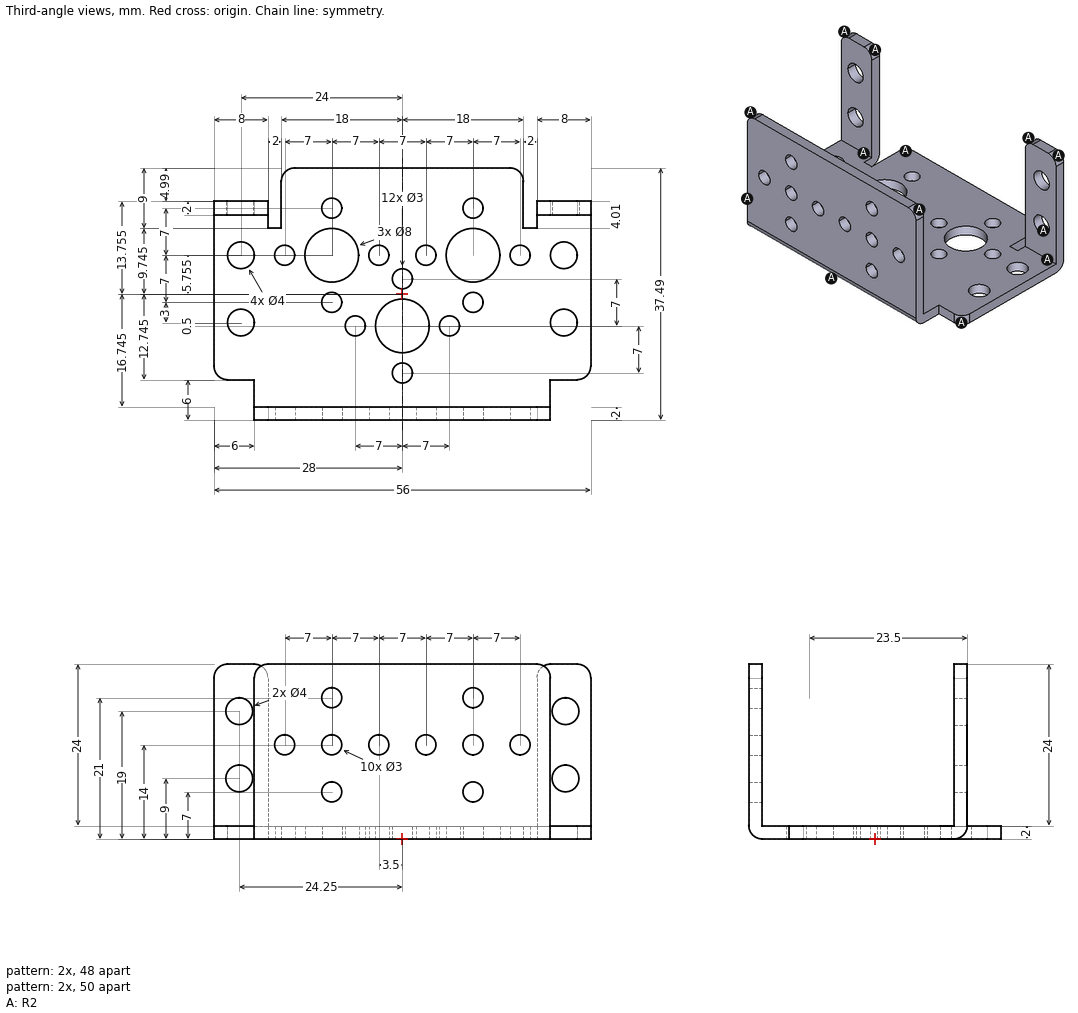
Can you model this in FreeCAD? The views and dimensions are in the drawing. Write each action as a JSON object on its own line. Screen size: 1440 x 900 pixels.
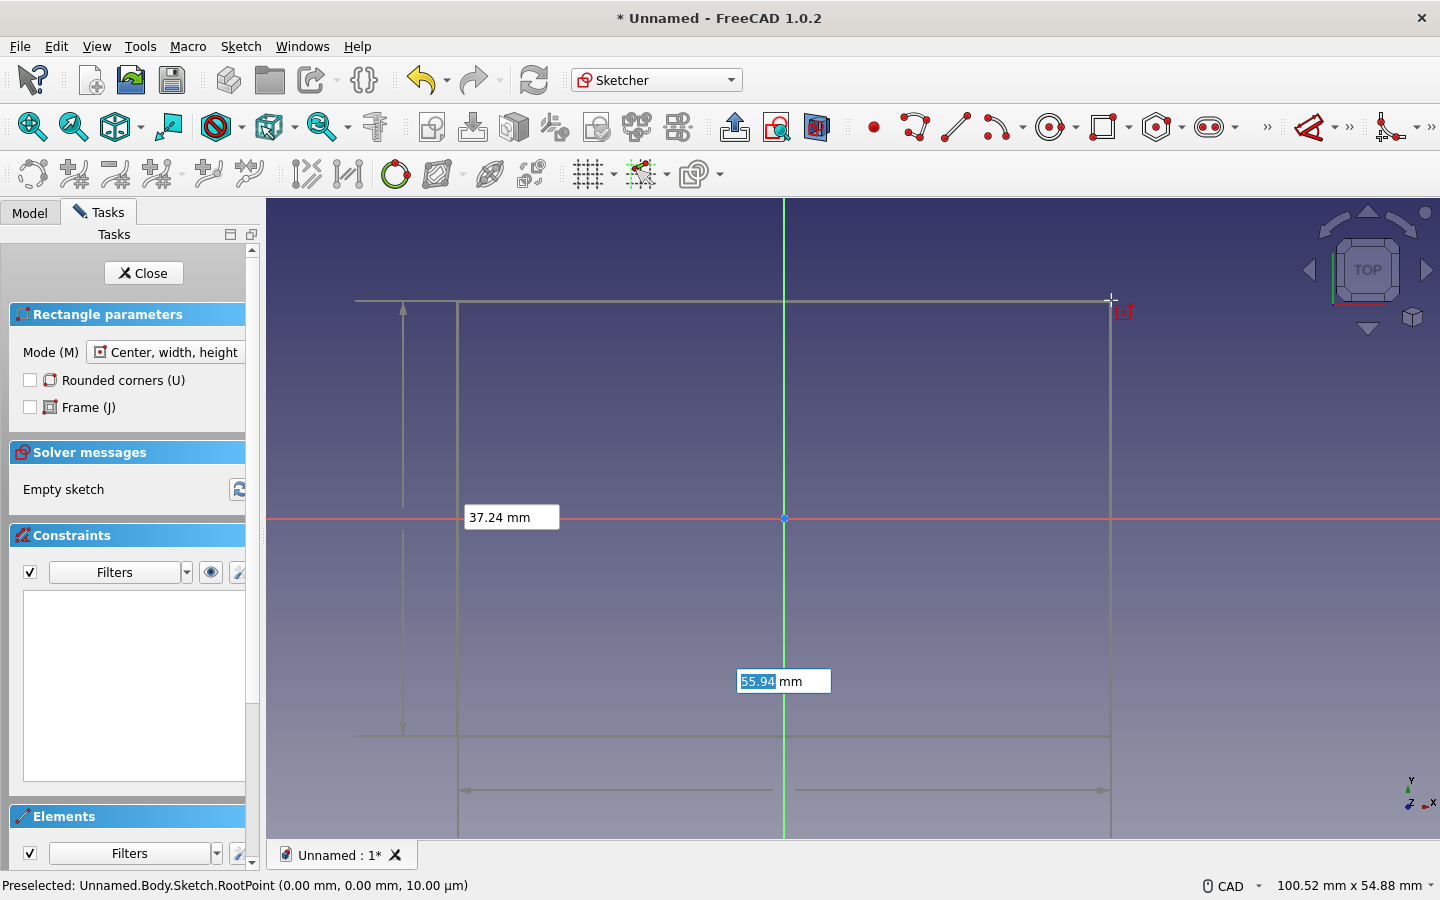
{"action": "type", "text": "56"}
{"action": "key", "text": "Tab"}
{"action": "type", "text": "37.49"}
{"action": "key", "text": "Return"}
{"action": "key", "text": "Escape"}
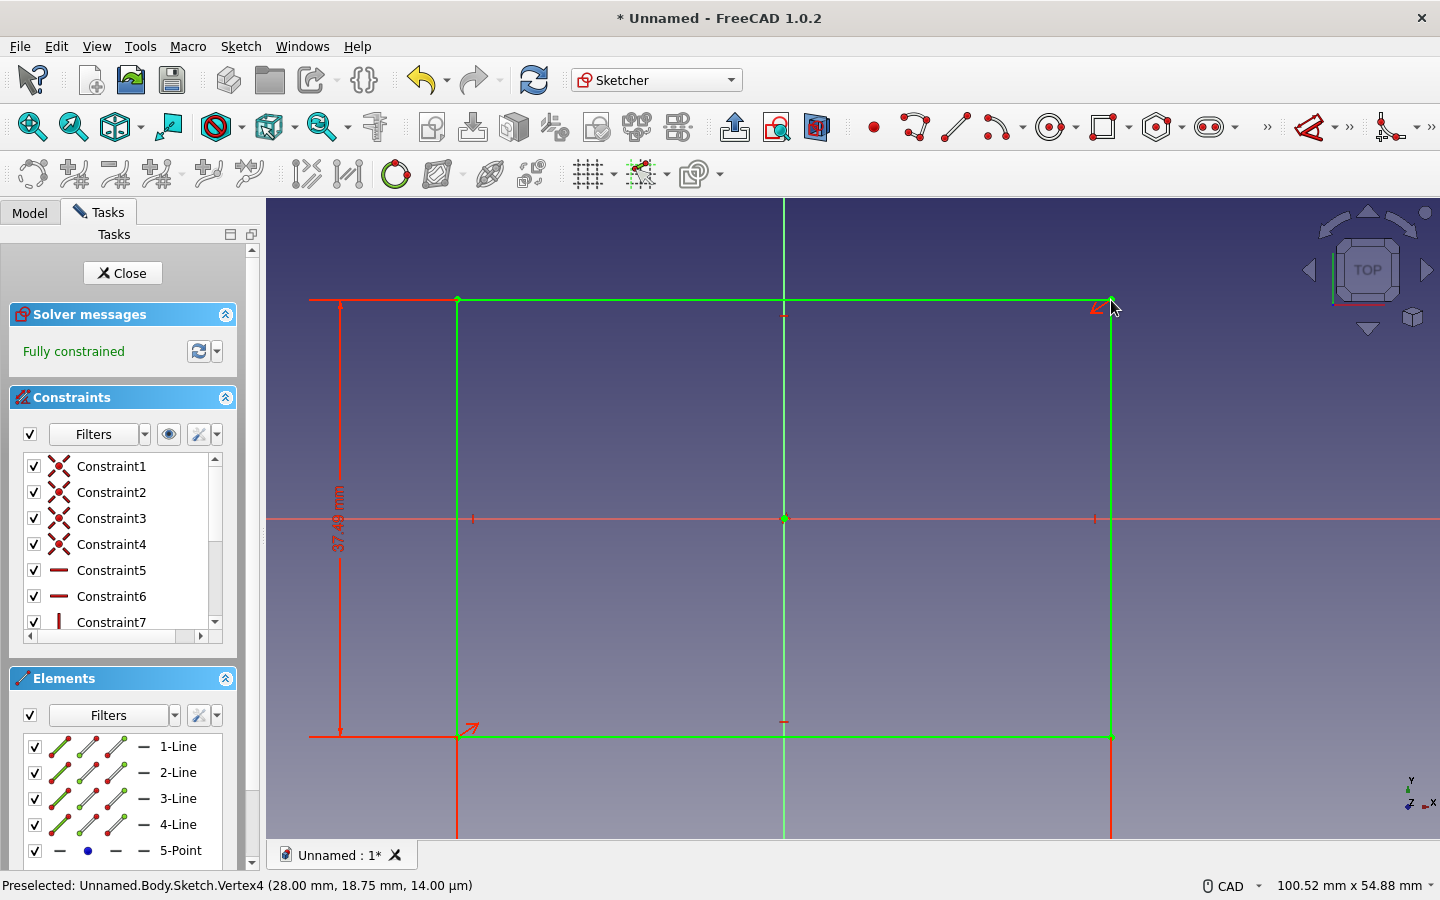
{"action": "left_click", "coordinate": [123, 273]}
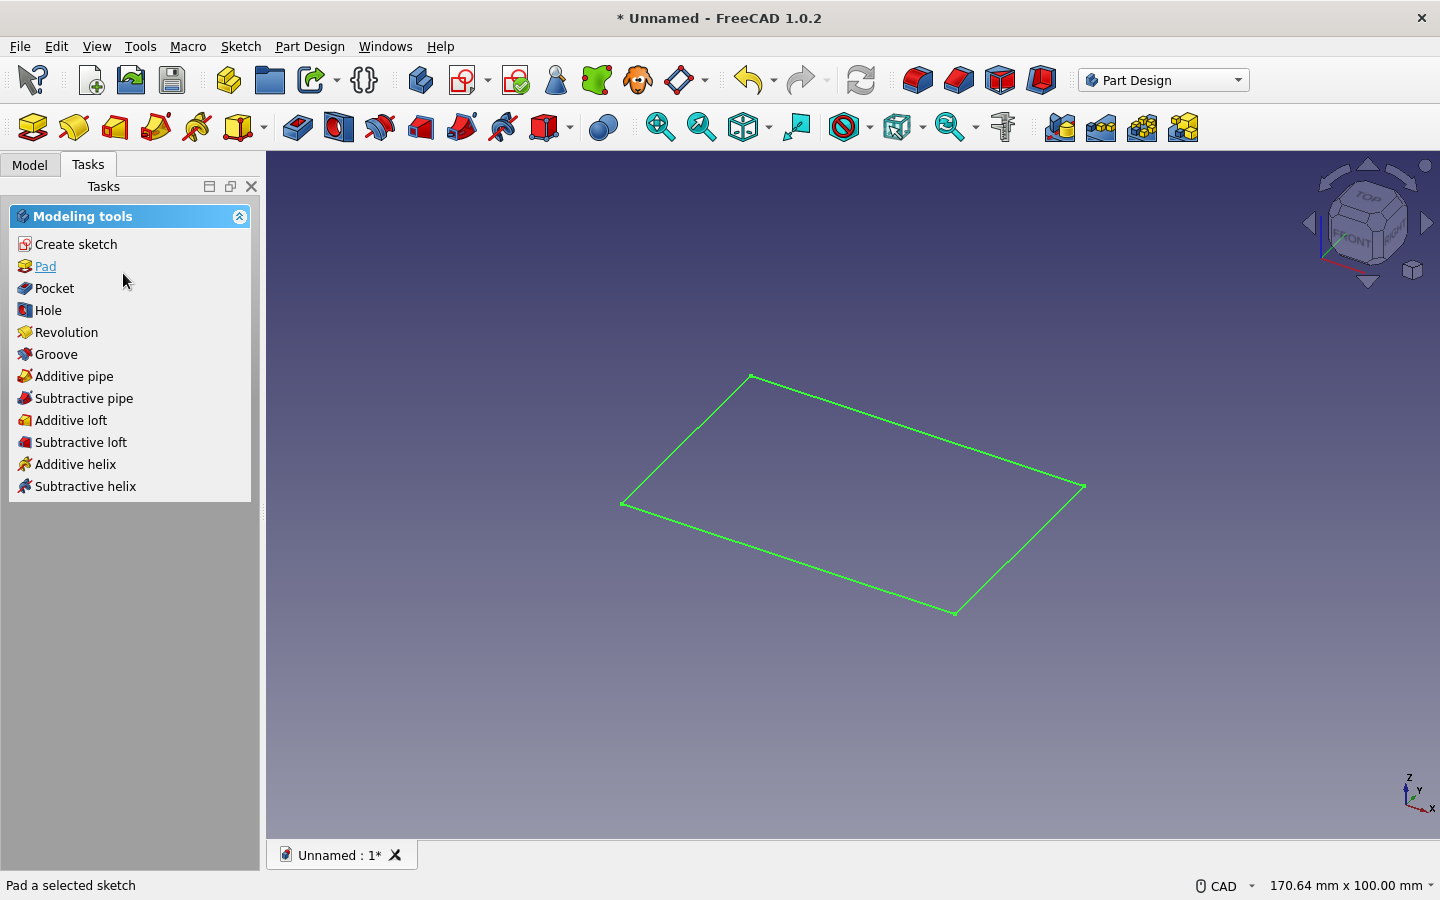
{"action": "left_click", "coordinate": [33, 128]}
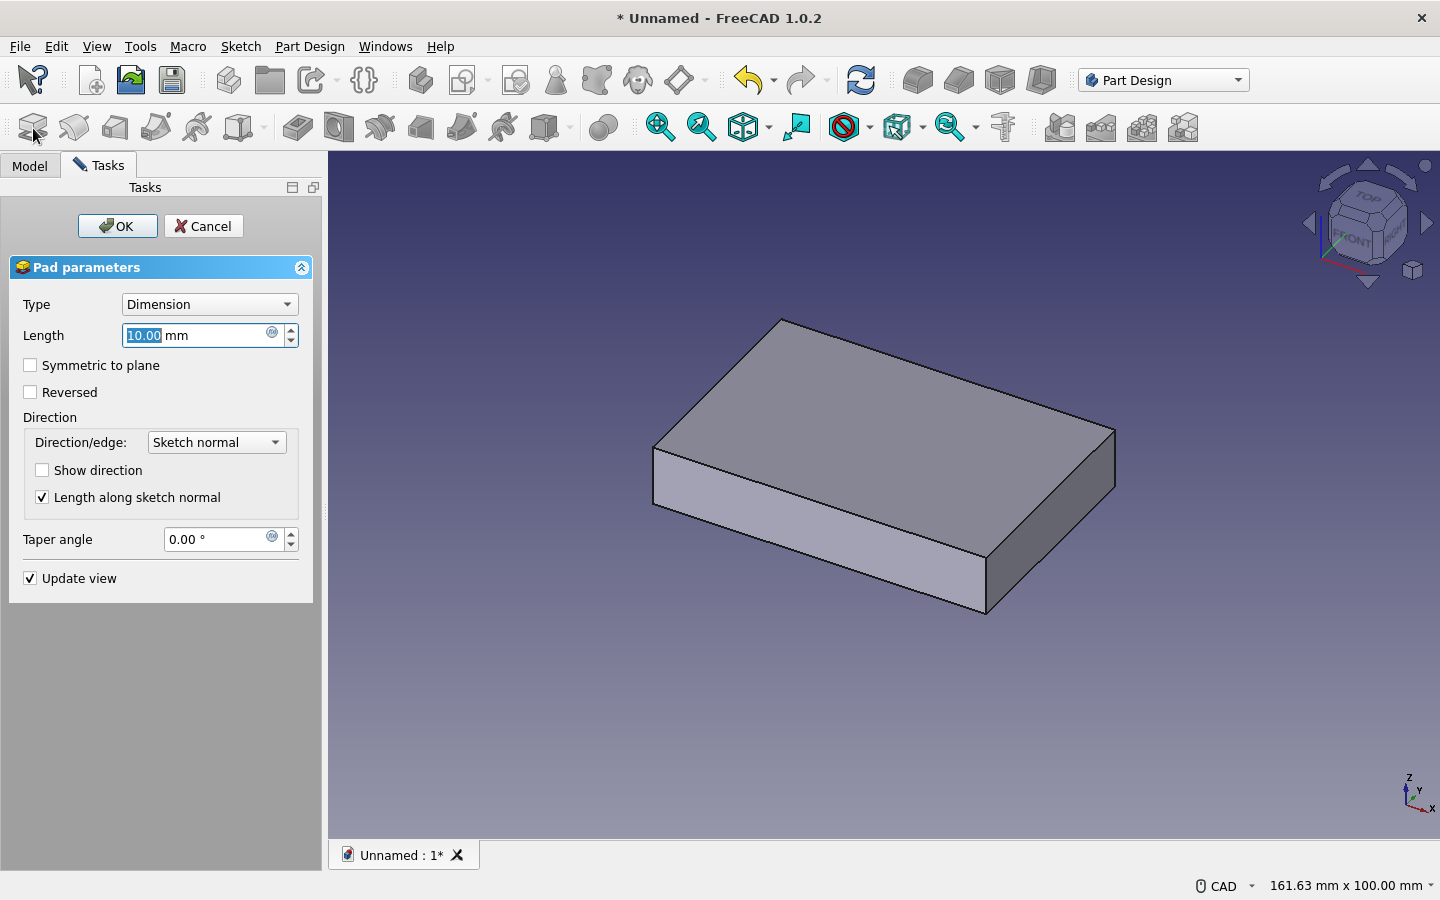
{"action": "type", "text": "2"}
{"action": "key", "text": "Tab"}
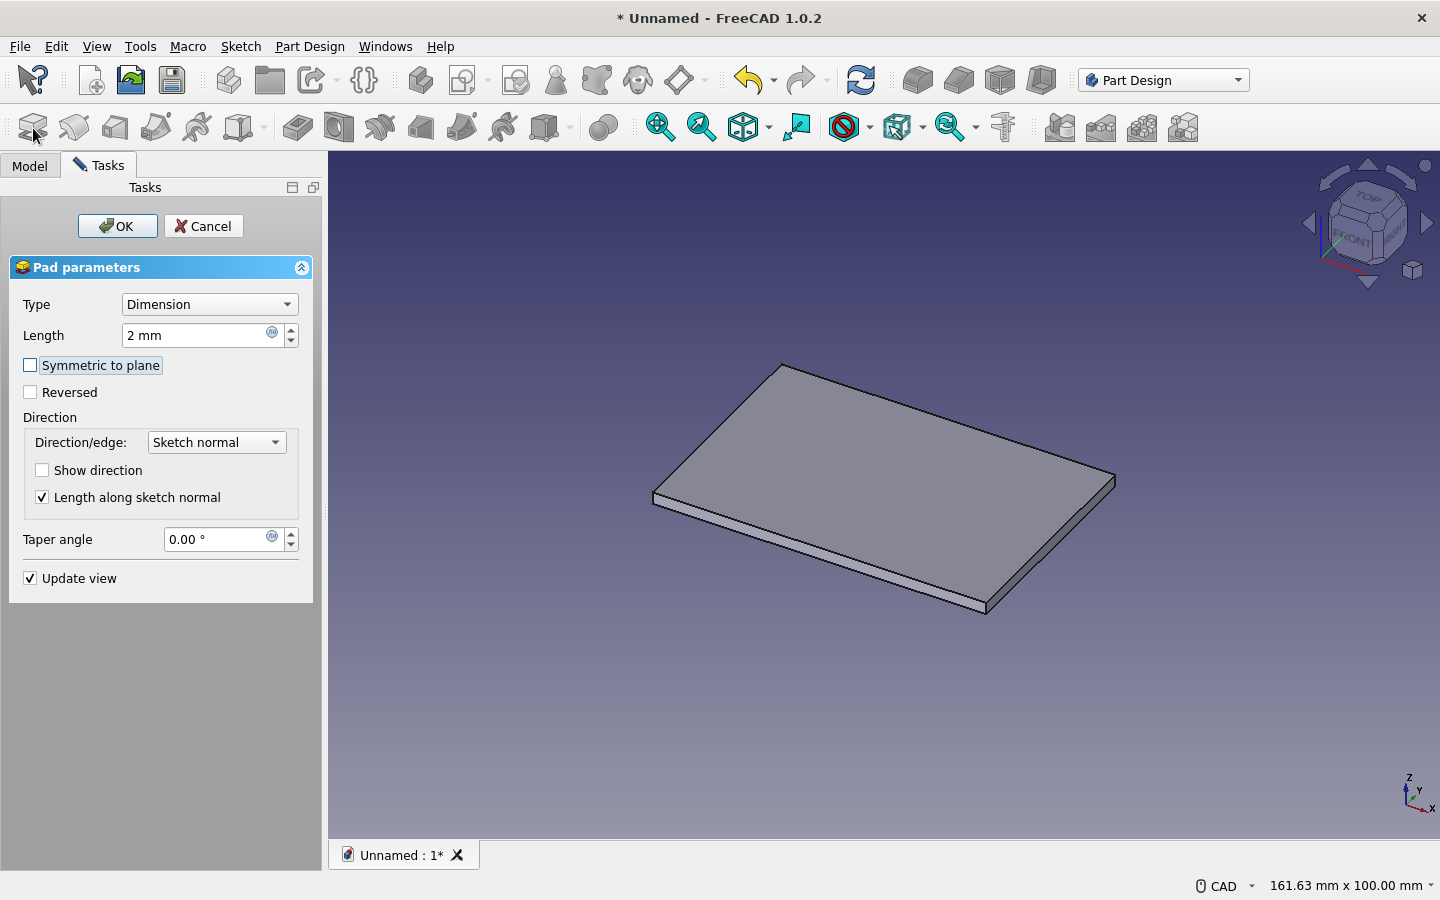
{"action": "left_click", "coordinate": [118, 226]}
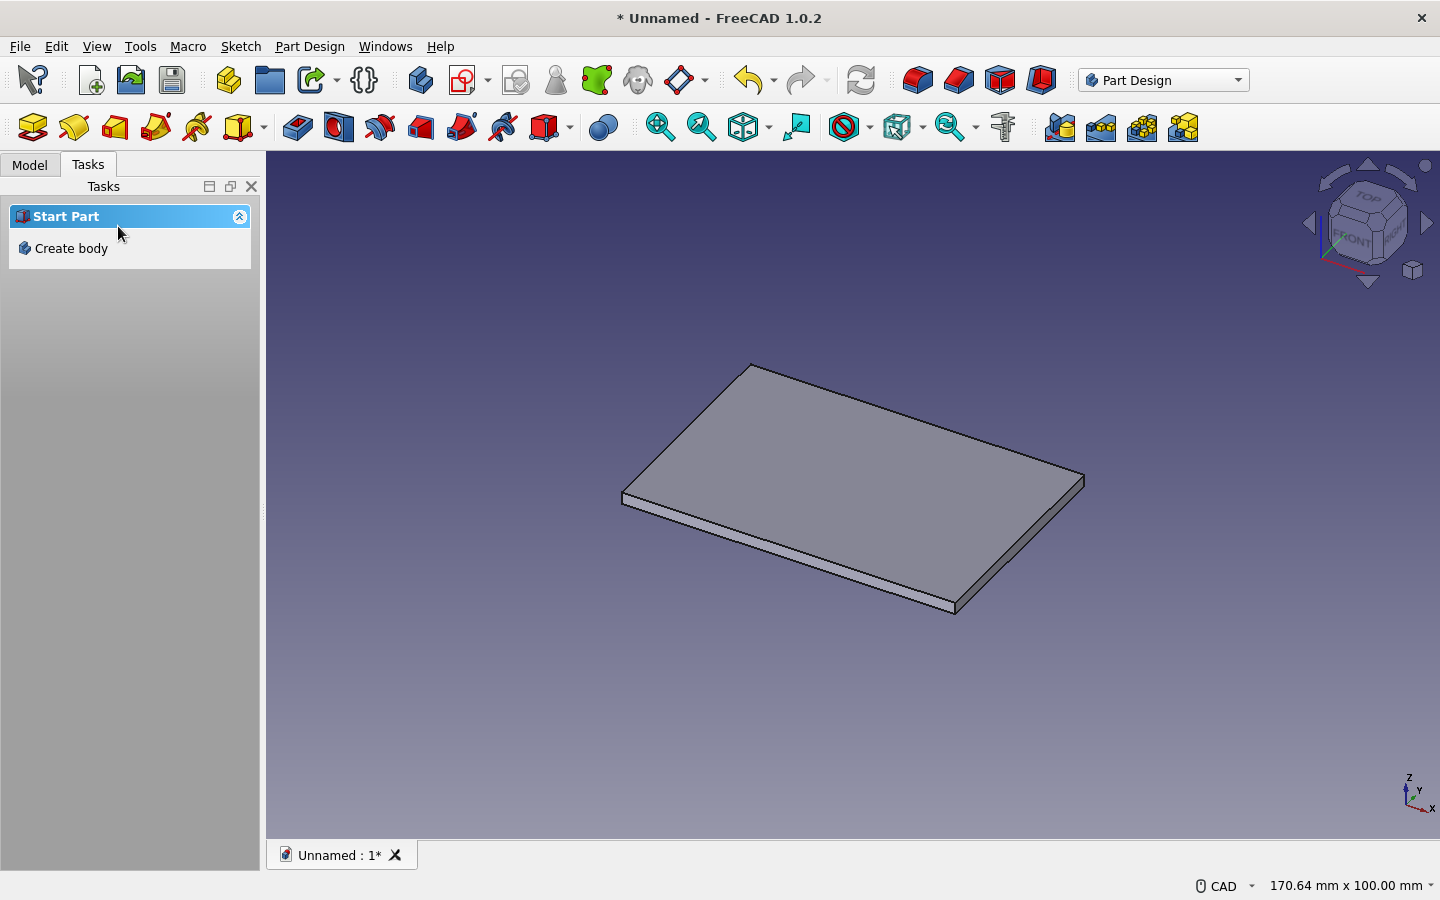
{"action": "left_click", "coordinate": [661, 128]}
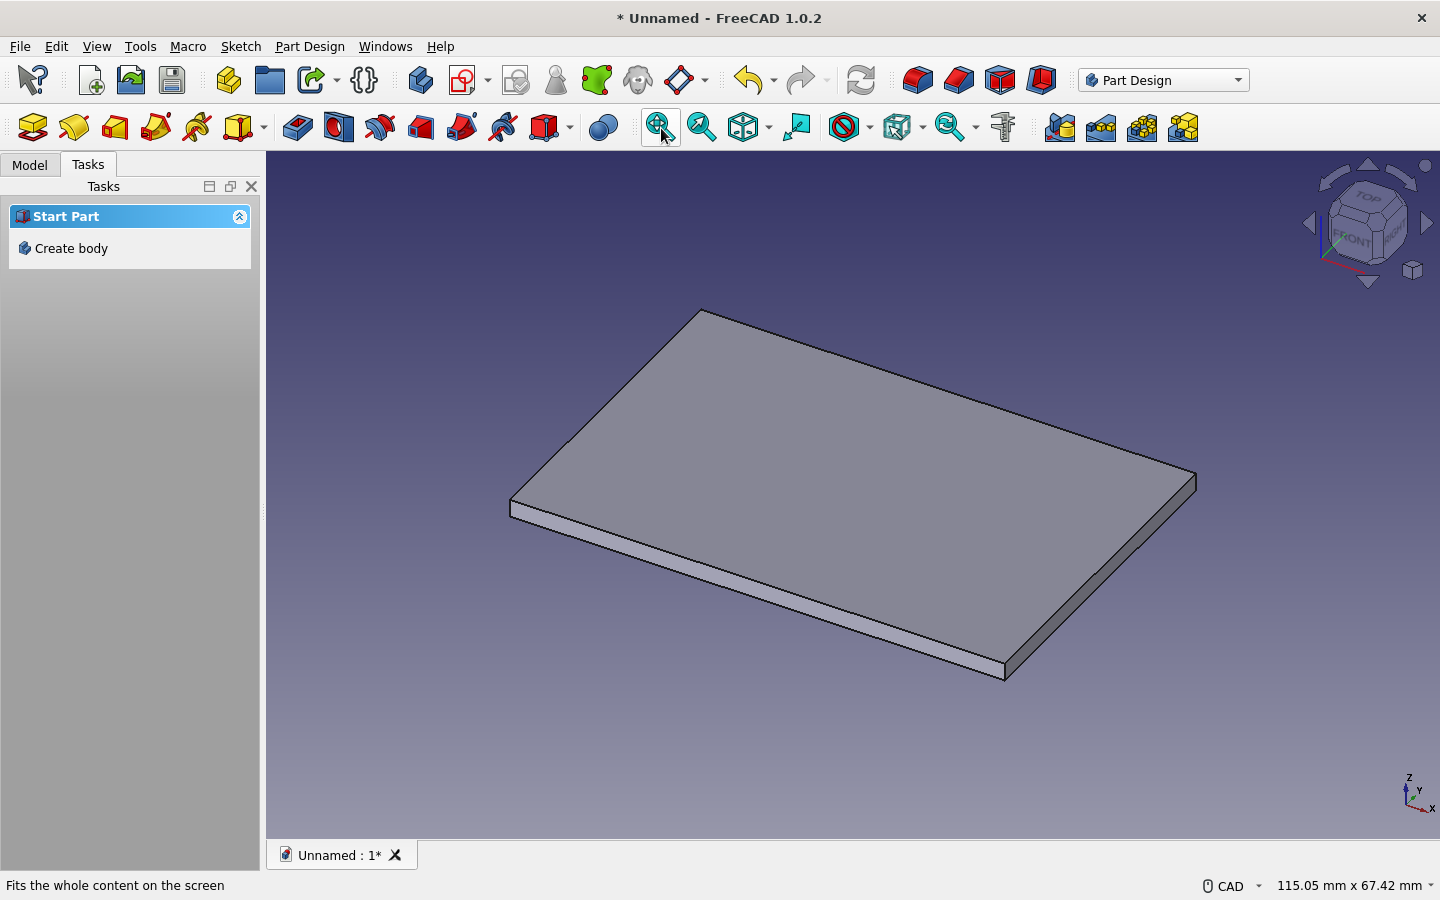
{"action": "left_click", "coordinate": [924, 509]}